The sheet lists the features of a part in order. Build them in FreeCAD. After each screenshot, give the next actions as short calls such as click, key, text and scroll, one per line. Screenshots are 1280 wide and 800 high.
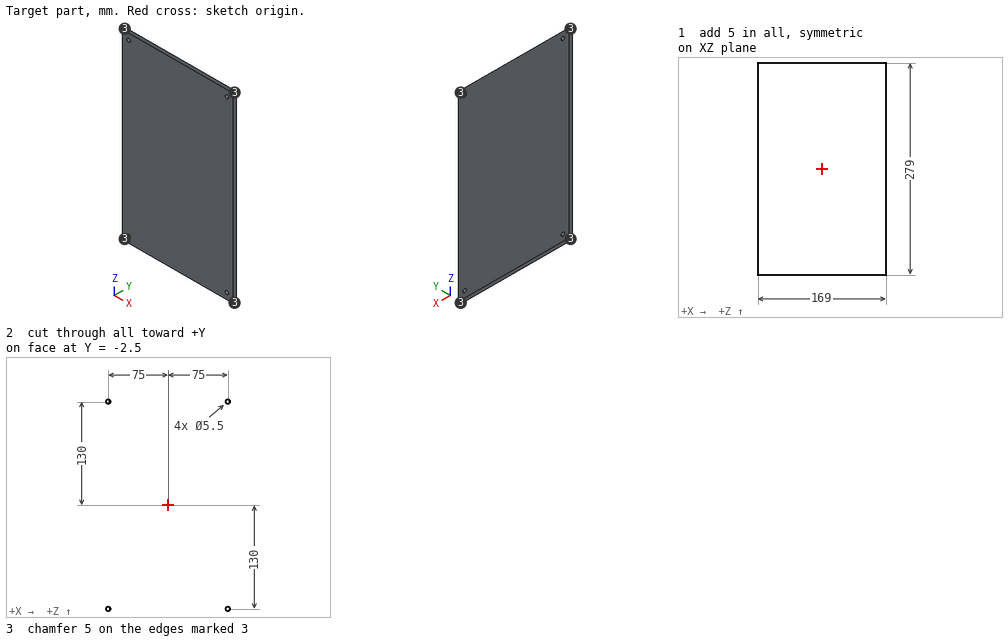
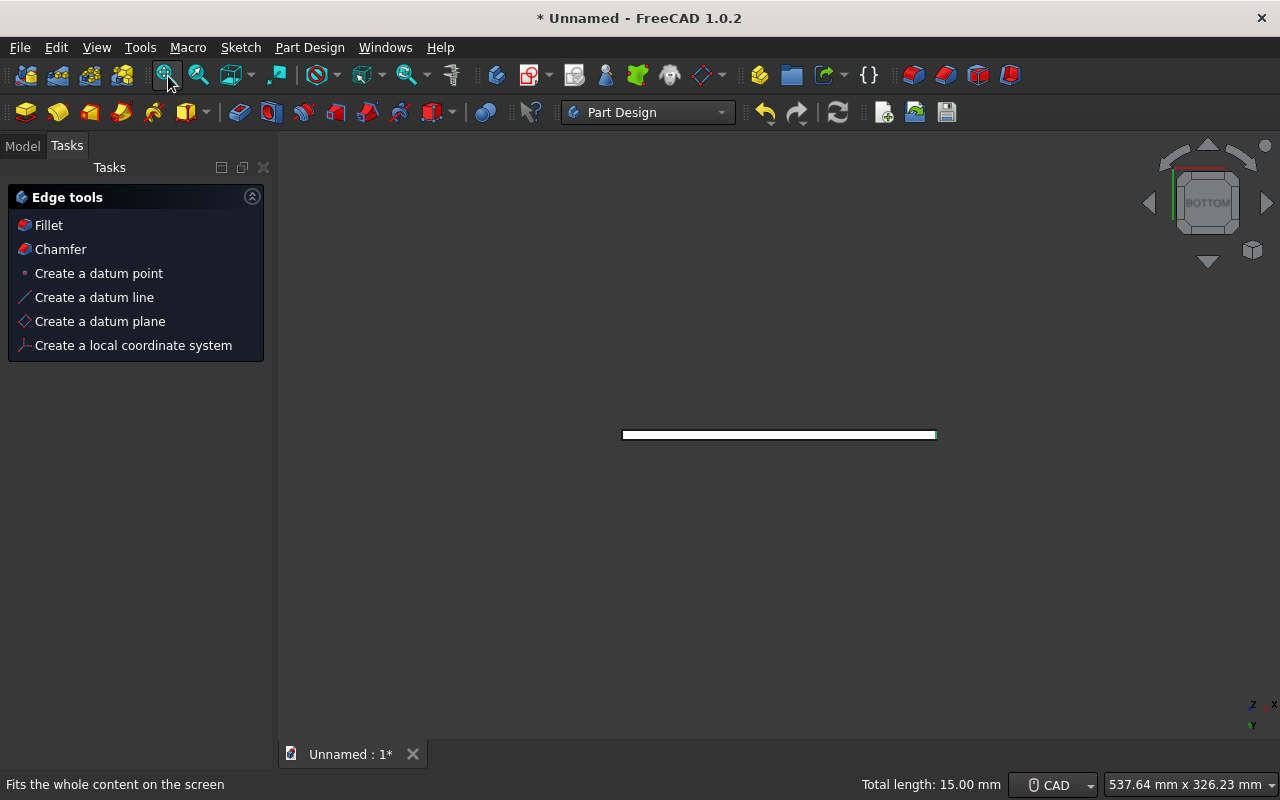
click(622, 436, ctrl)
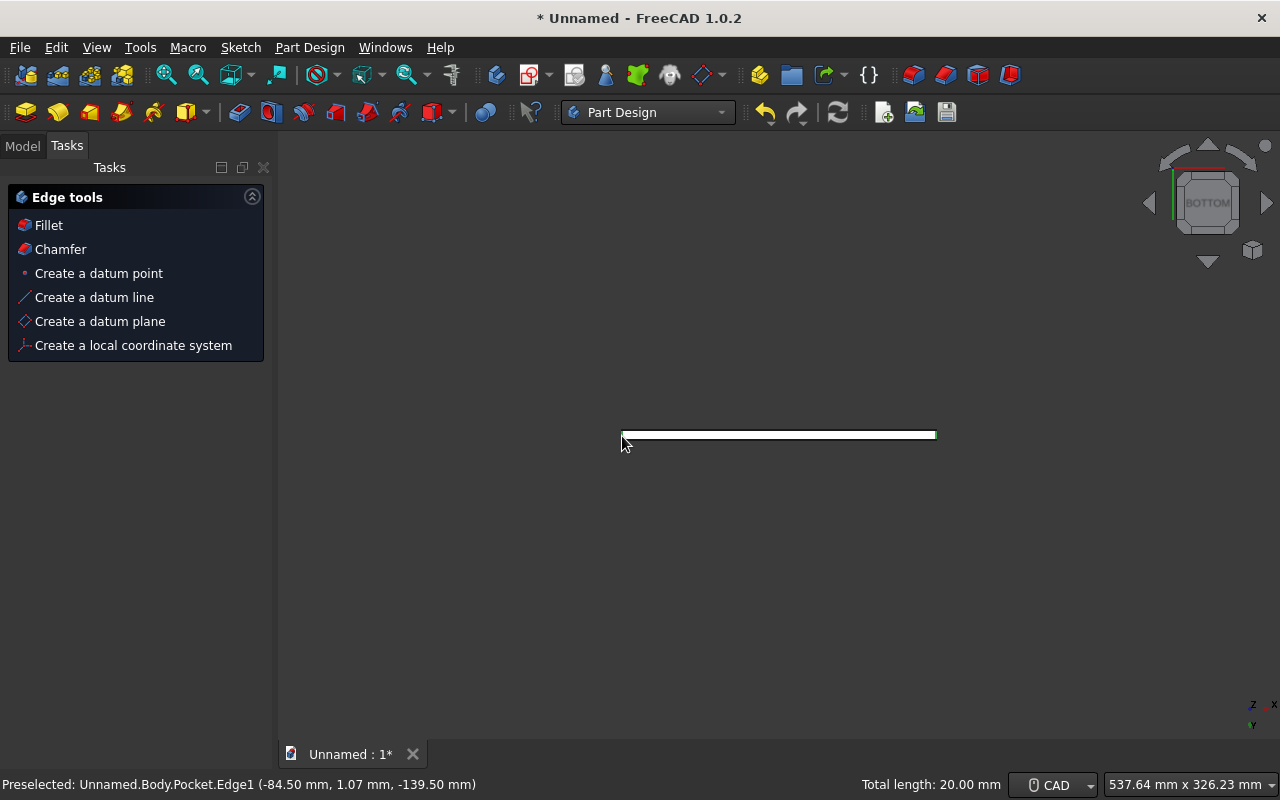
click(946, 76)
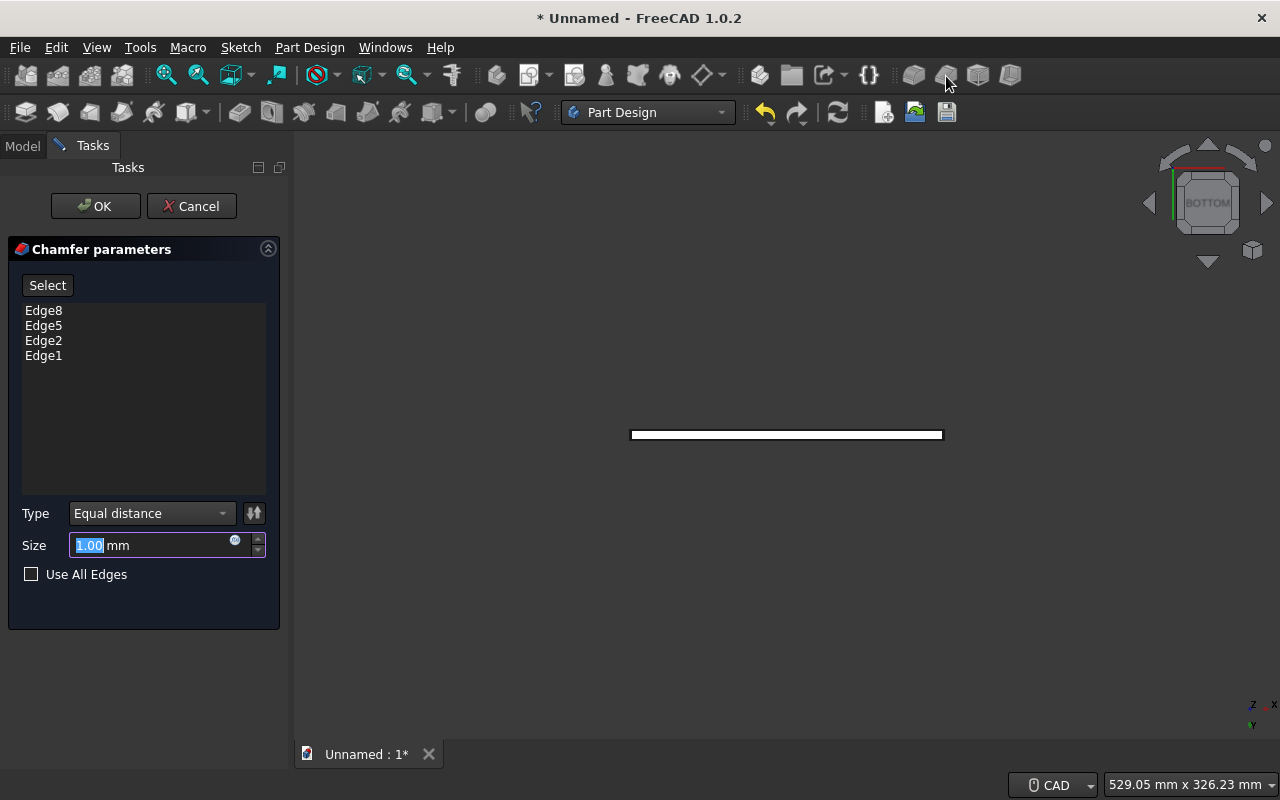
text(5)
key(Tab)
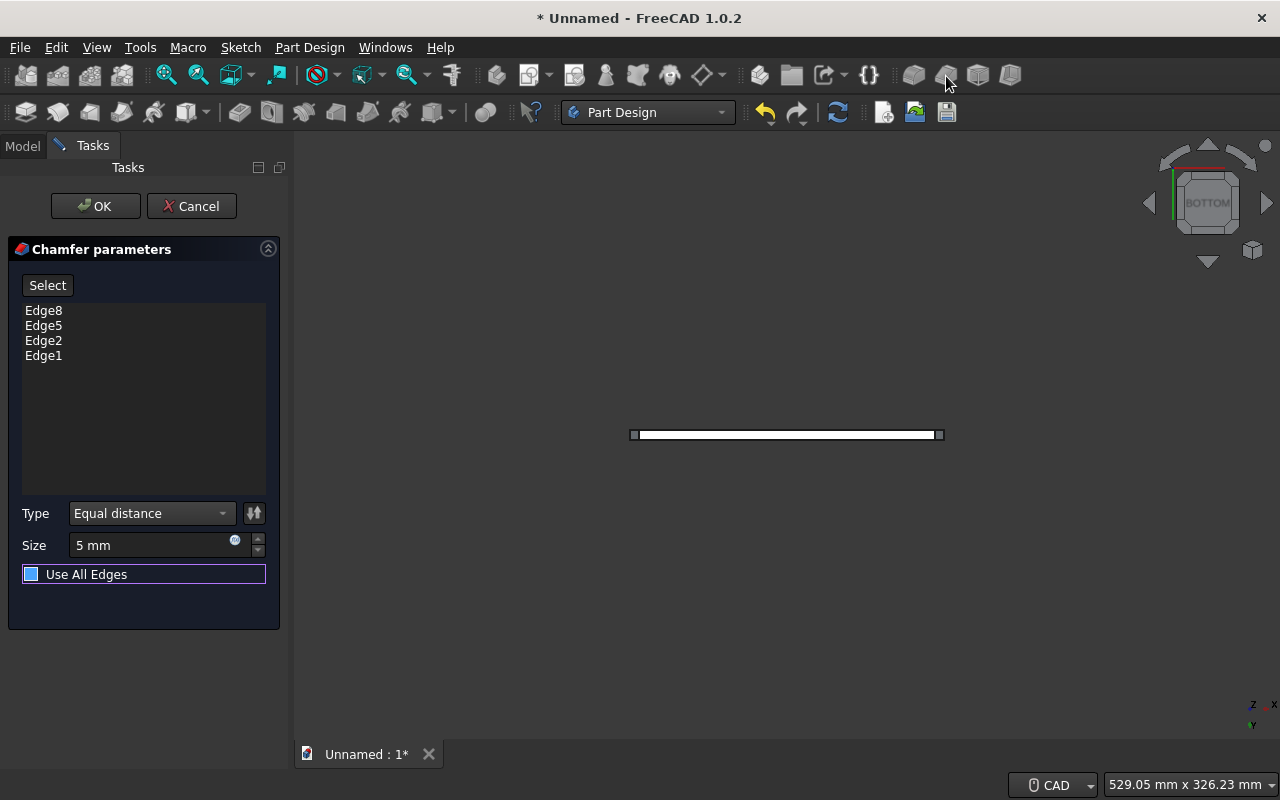
click(96, 206)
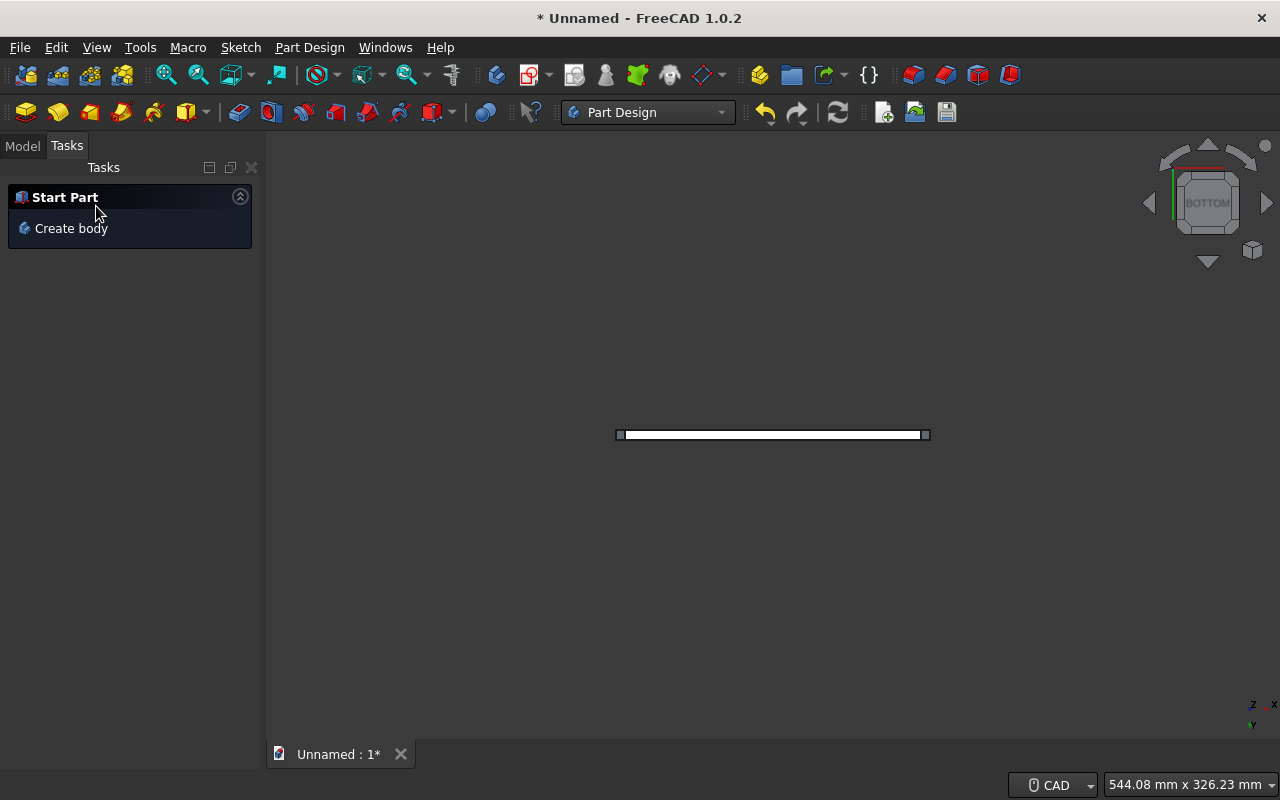
key(0)